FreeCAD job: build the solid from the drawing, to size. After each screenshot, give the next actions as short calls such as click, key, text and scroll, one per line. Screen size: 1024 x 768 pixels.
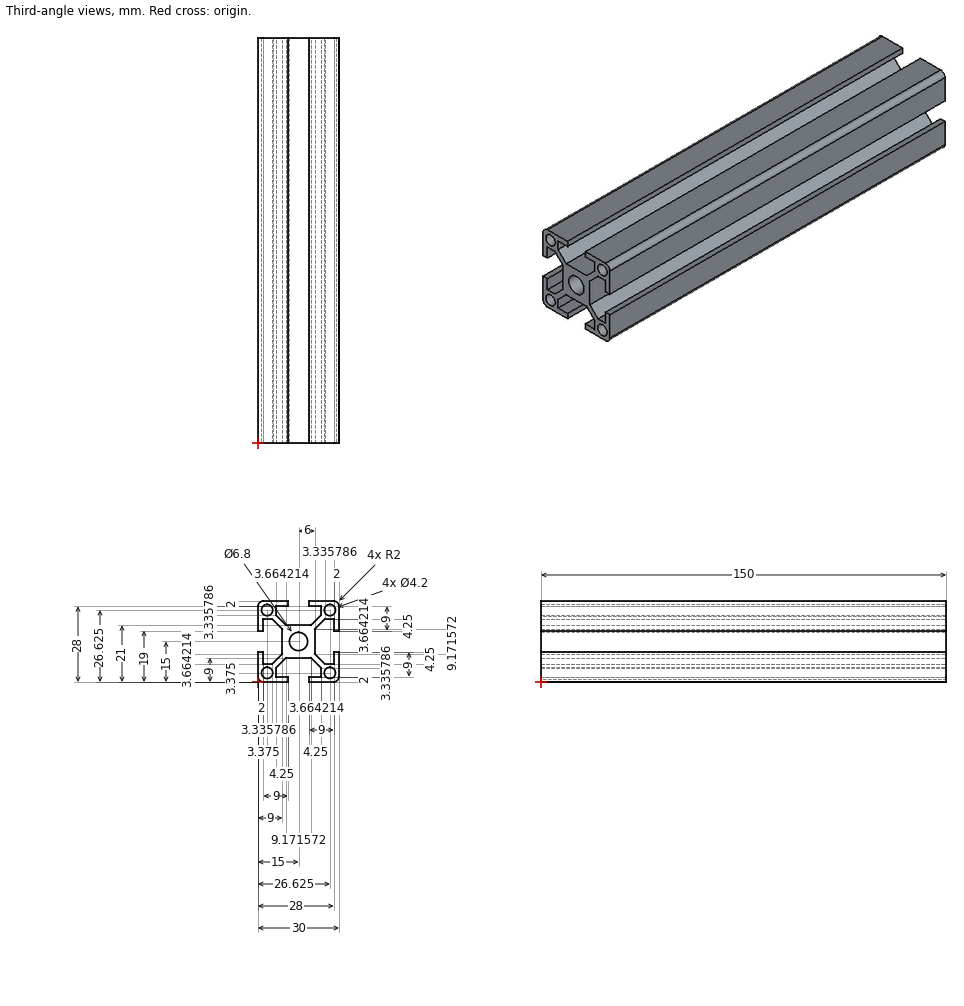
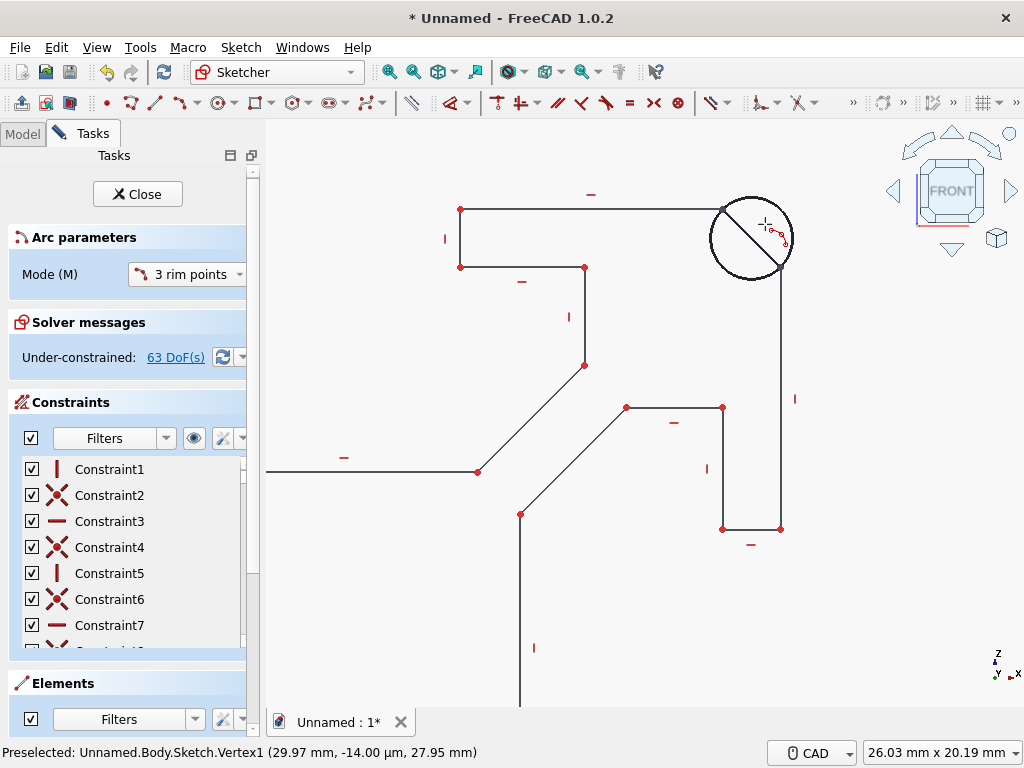
click(764, 225)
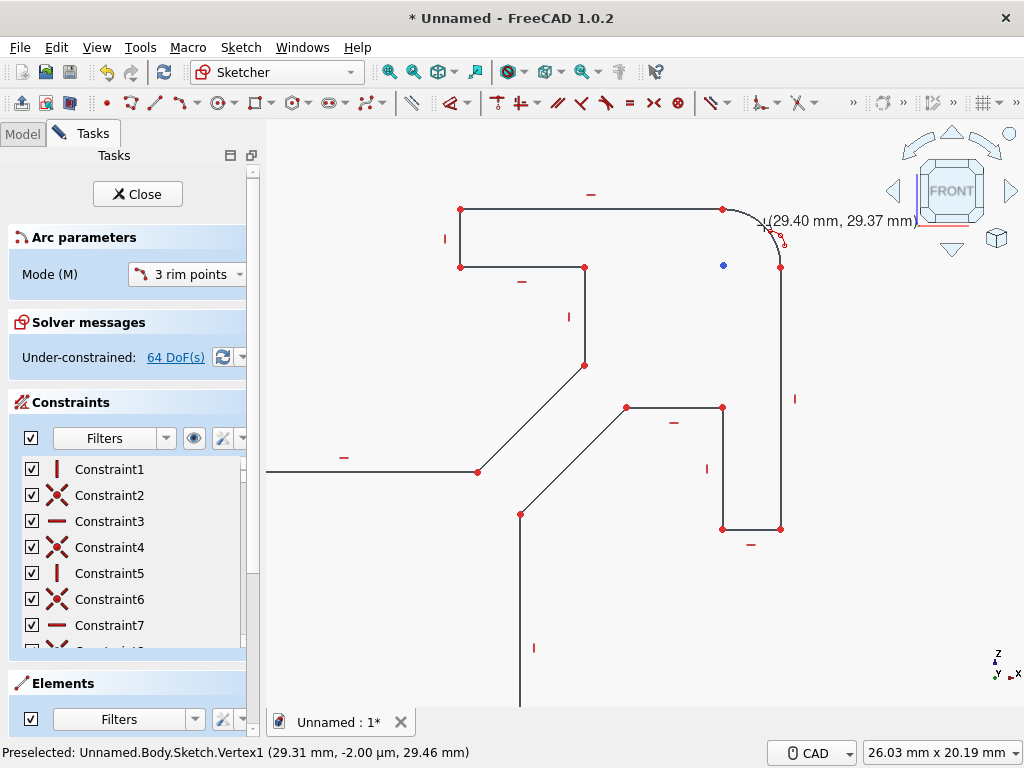
click(218, 104)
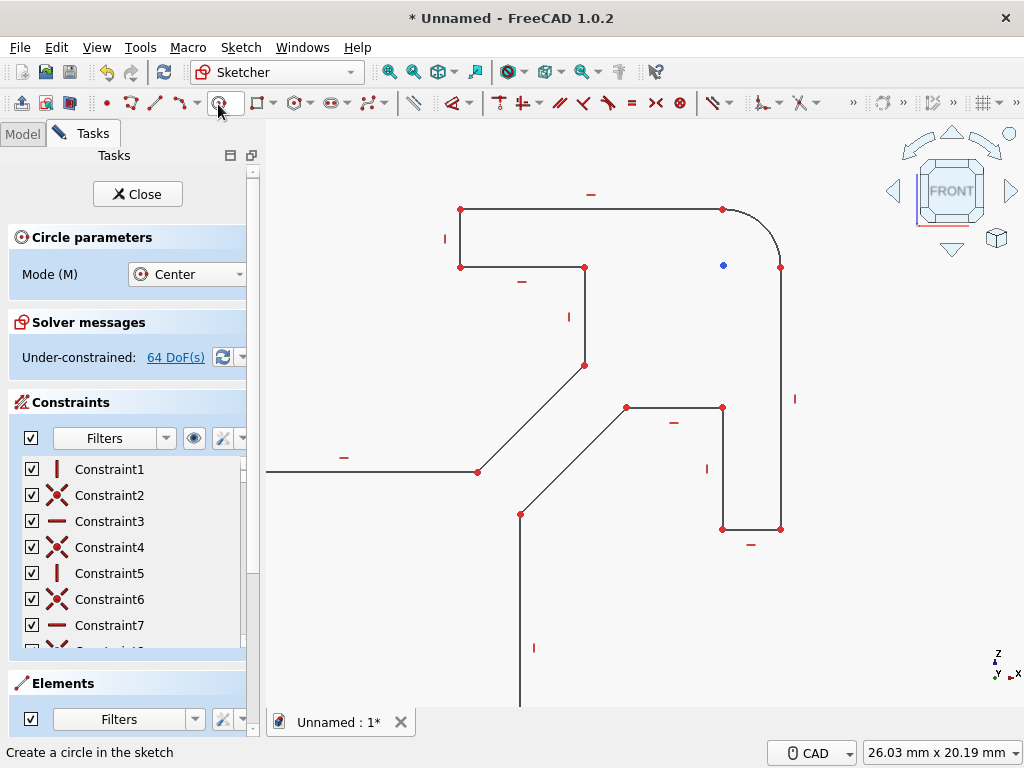
click(683, 306)
move(640, 263)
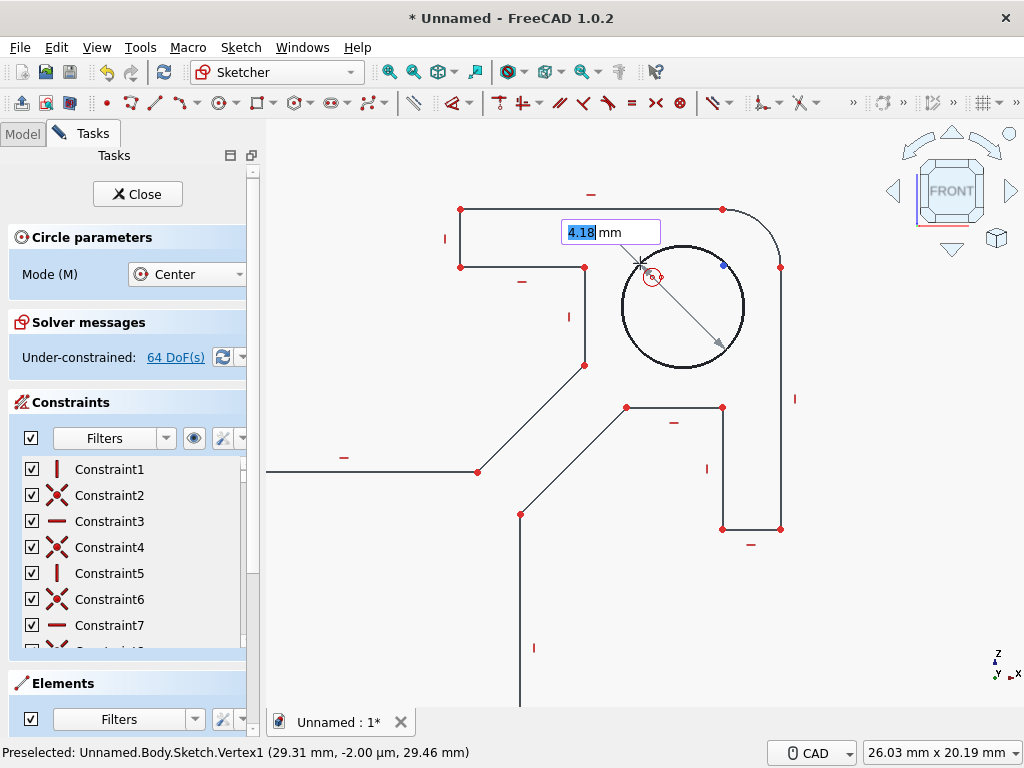
text(4.2)
key(Return)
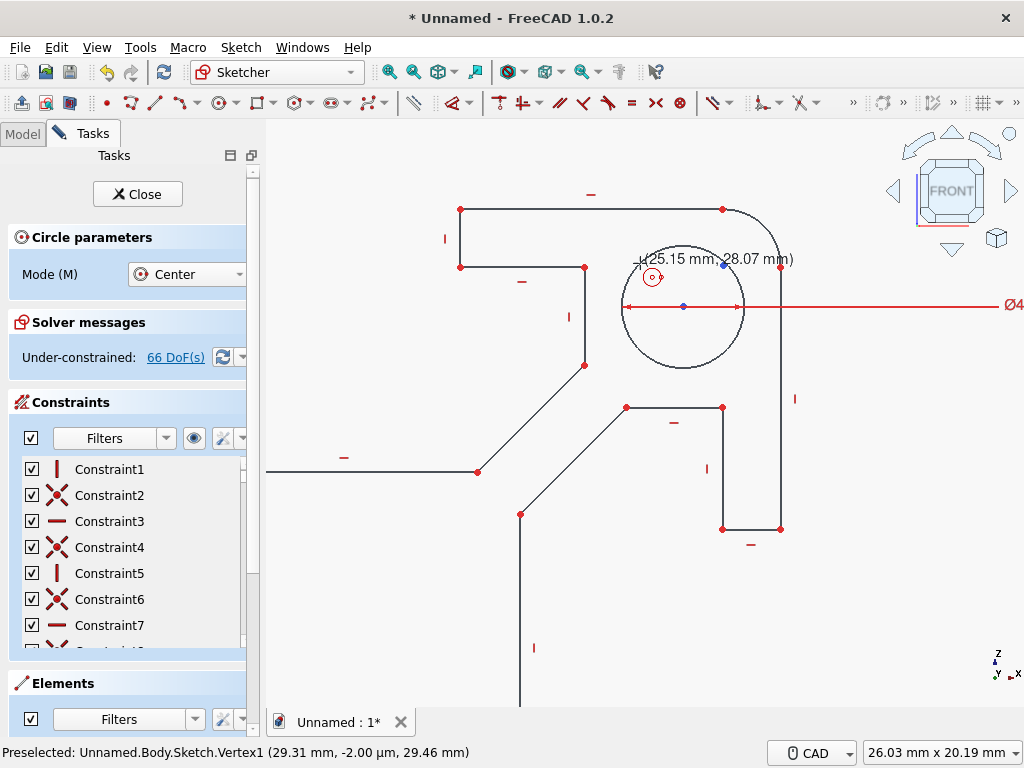
scroll(766, 224, down, 4)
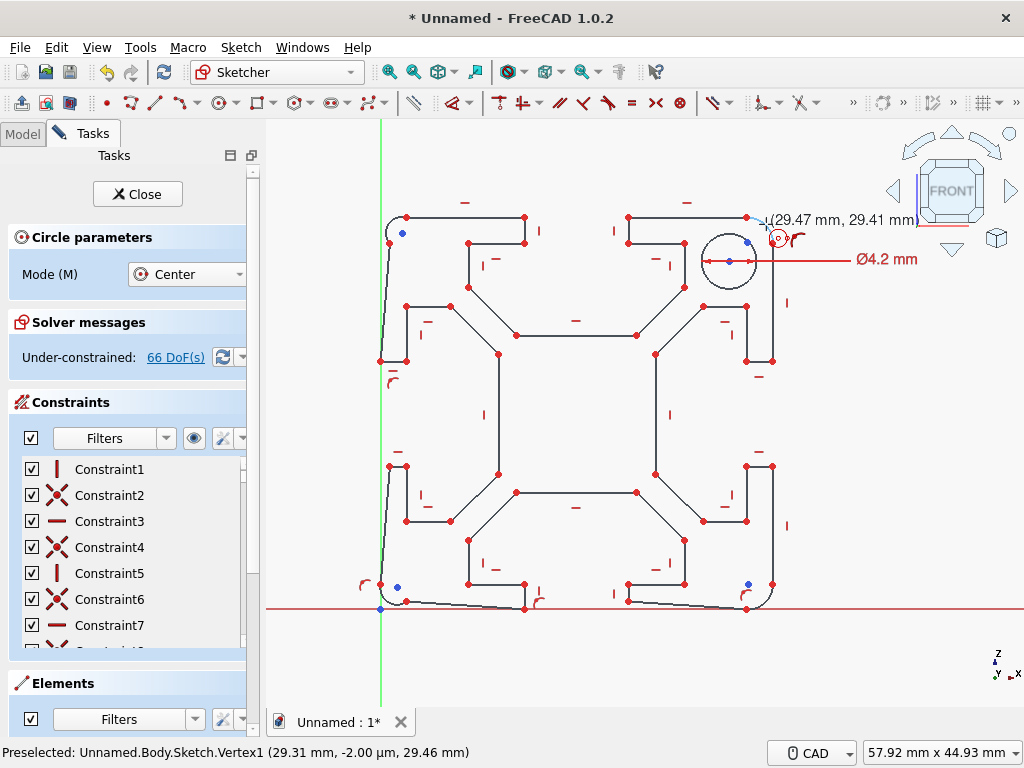
click(425, 261)
move(444, 242)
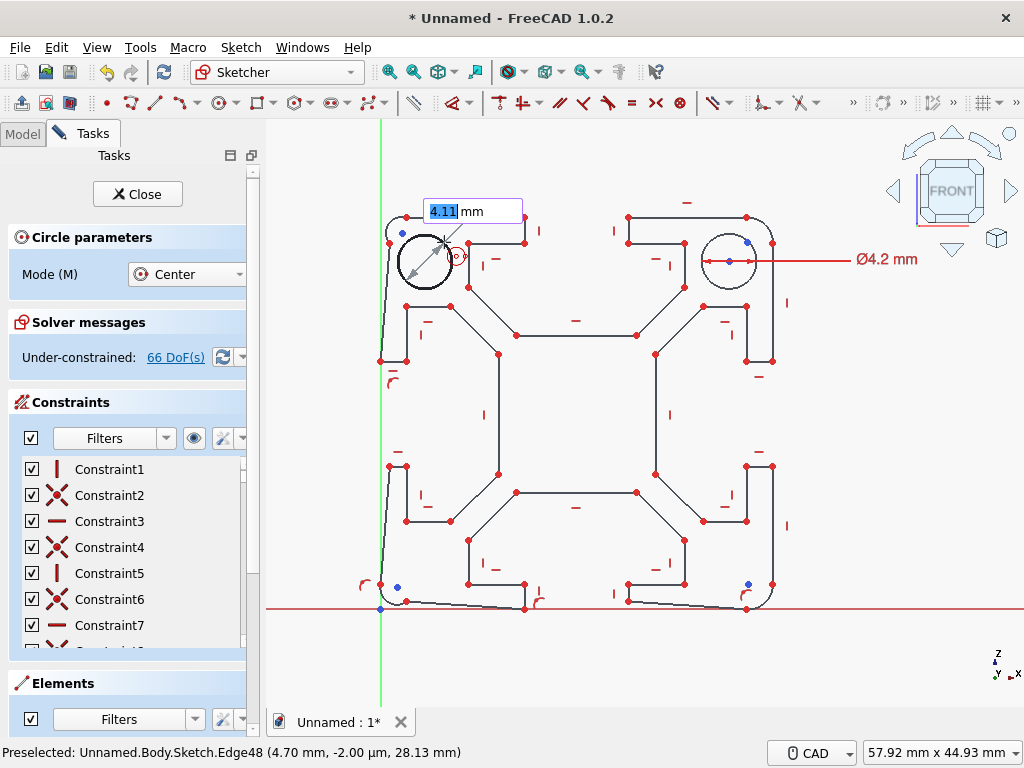
text(4.2)
key(Return)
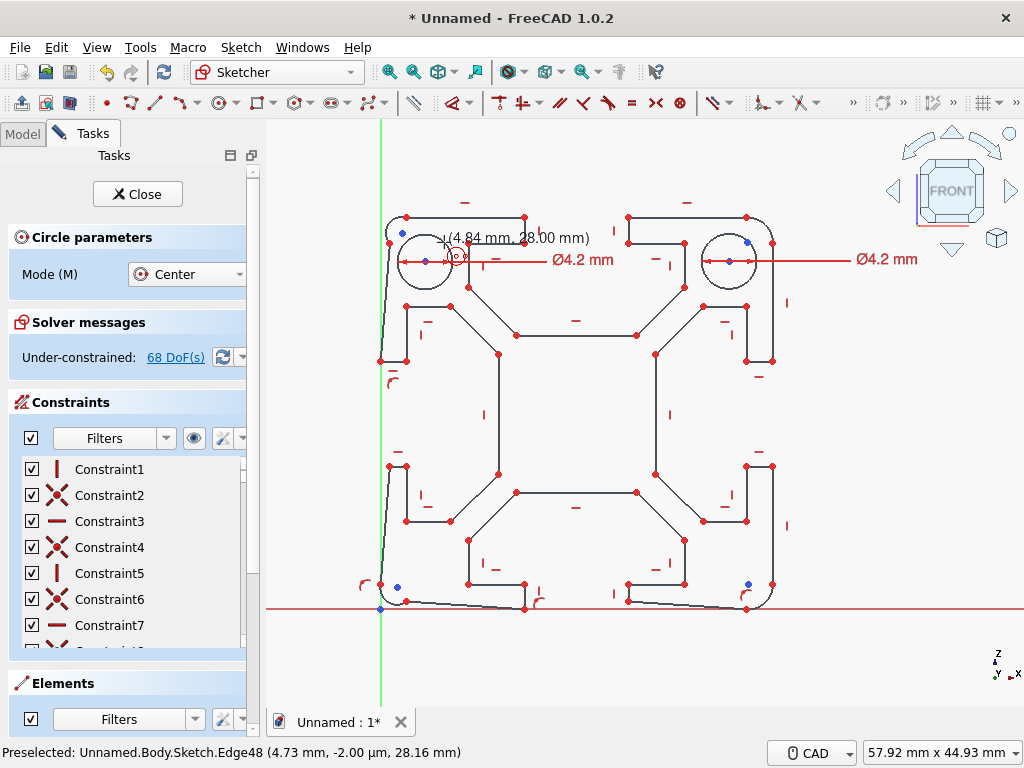
click(729, 565)
move(749, 546)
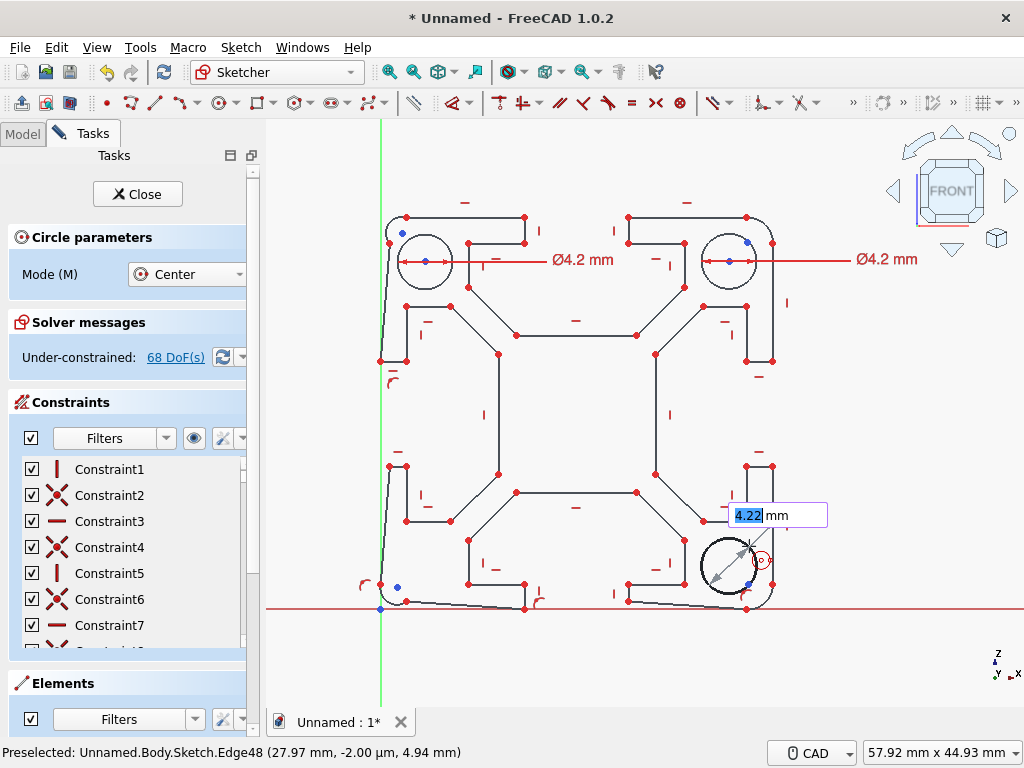
text(4.2)
key(Return)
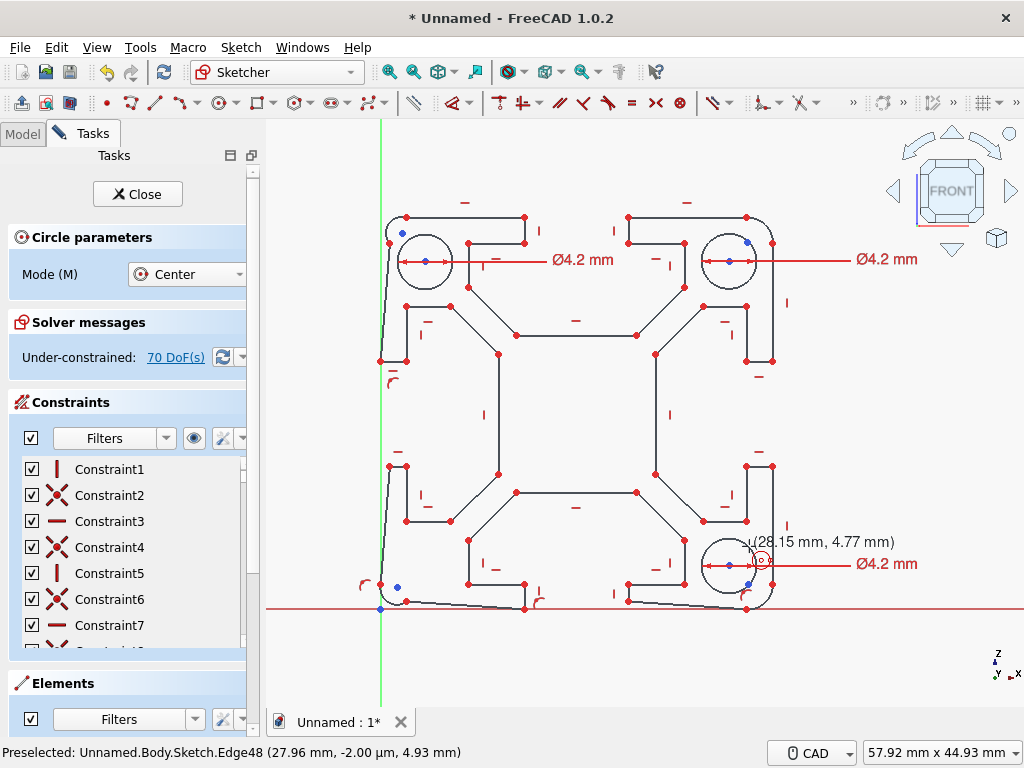
click(577, 413)
move(608, 382)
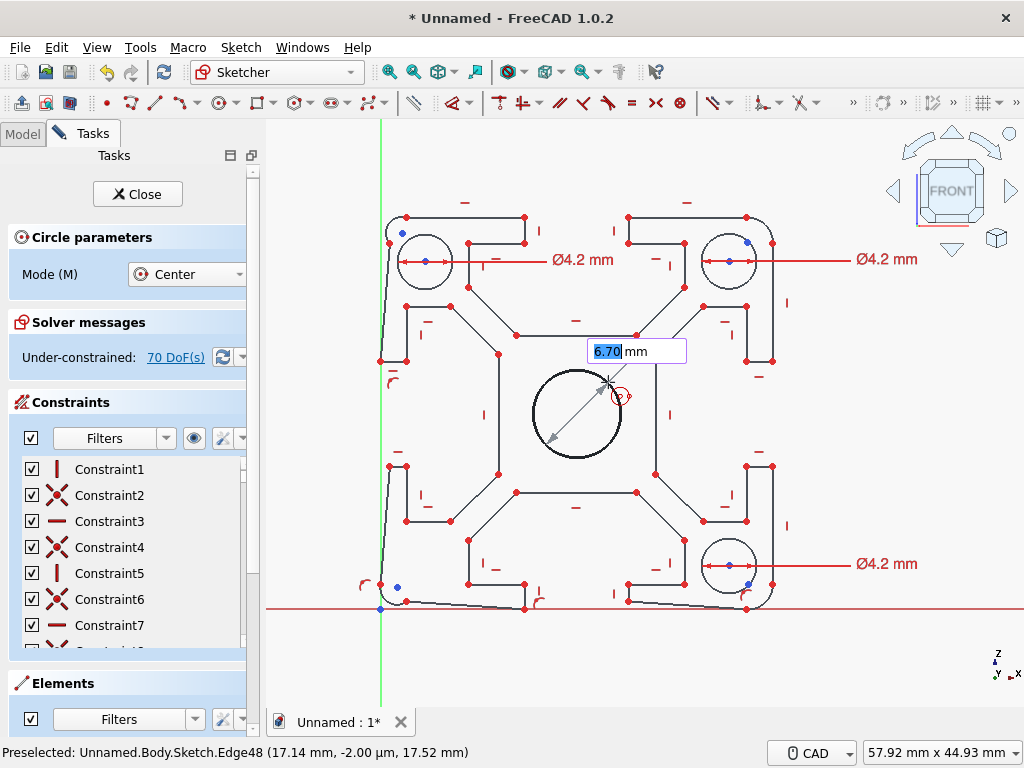
text(6.8)
key(Return)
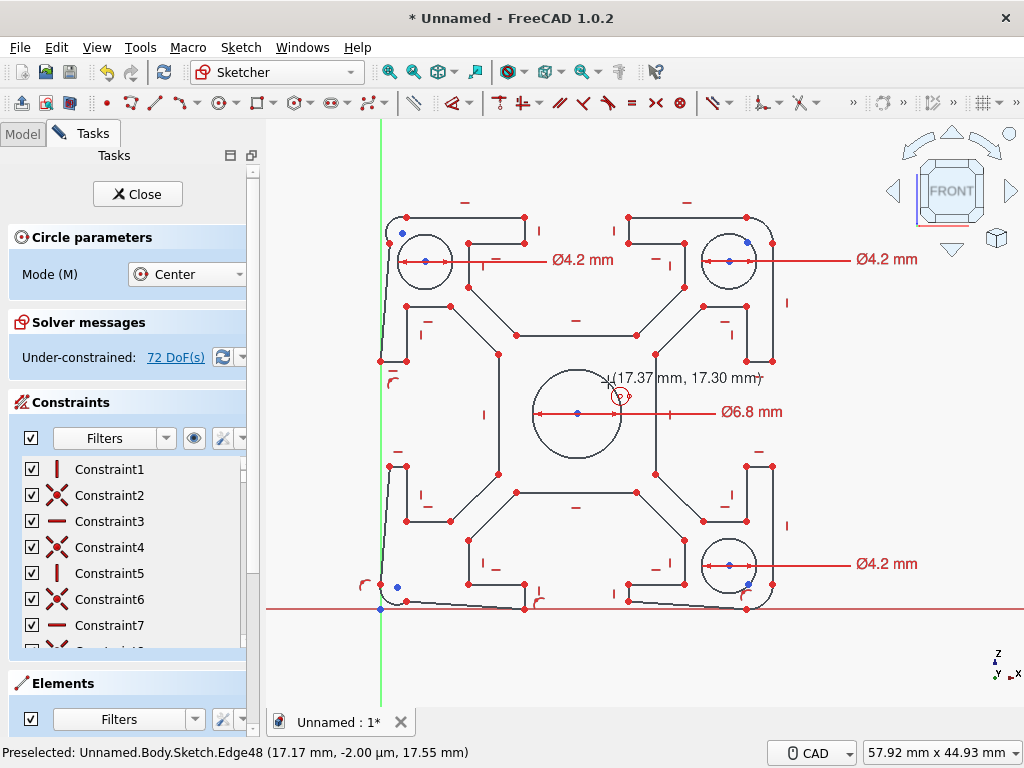
click(425, 565)
move(444, 546)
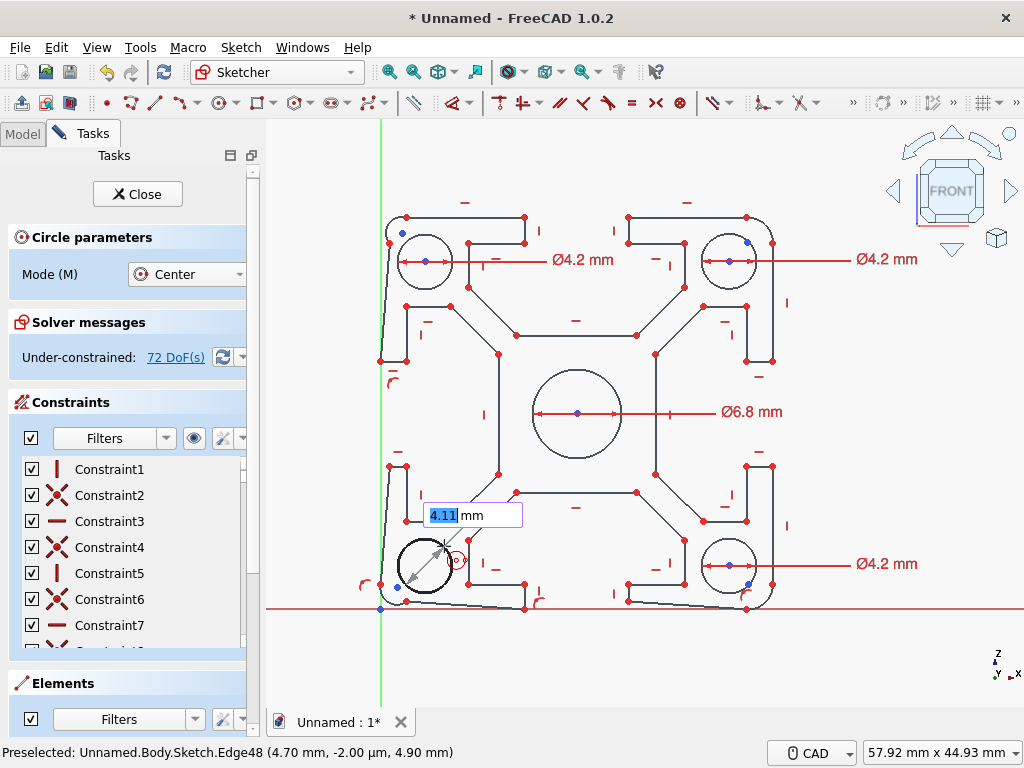
text(4.2)
key(Return)
key(Escape)